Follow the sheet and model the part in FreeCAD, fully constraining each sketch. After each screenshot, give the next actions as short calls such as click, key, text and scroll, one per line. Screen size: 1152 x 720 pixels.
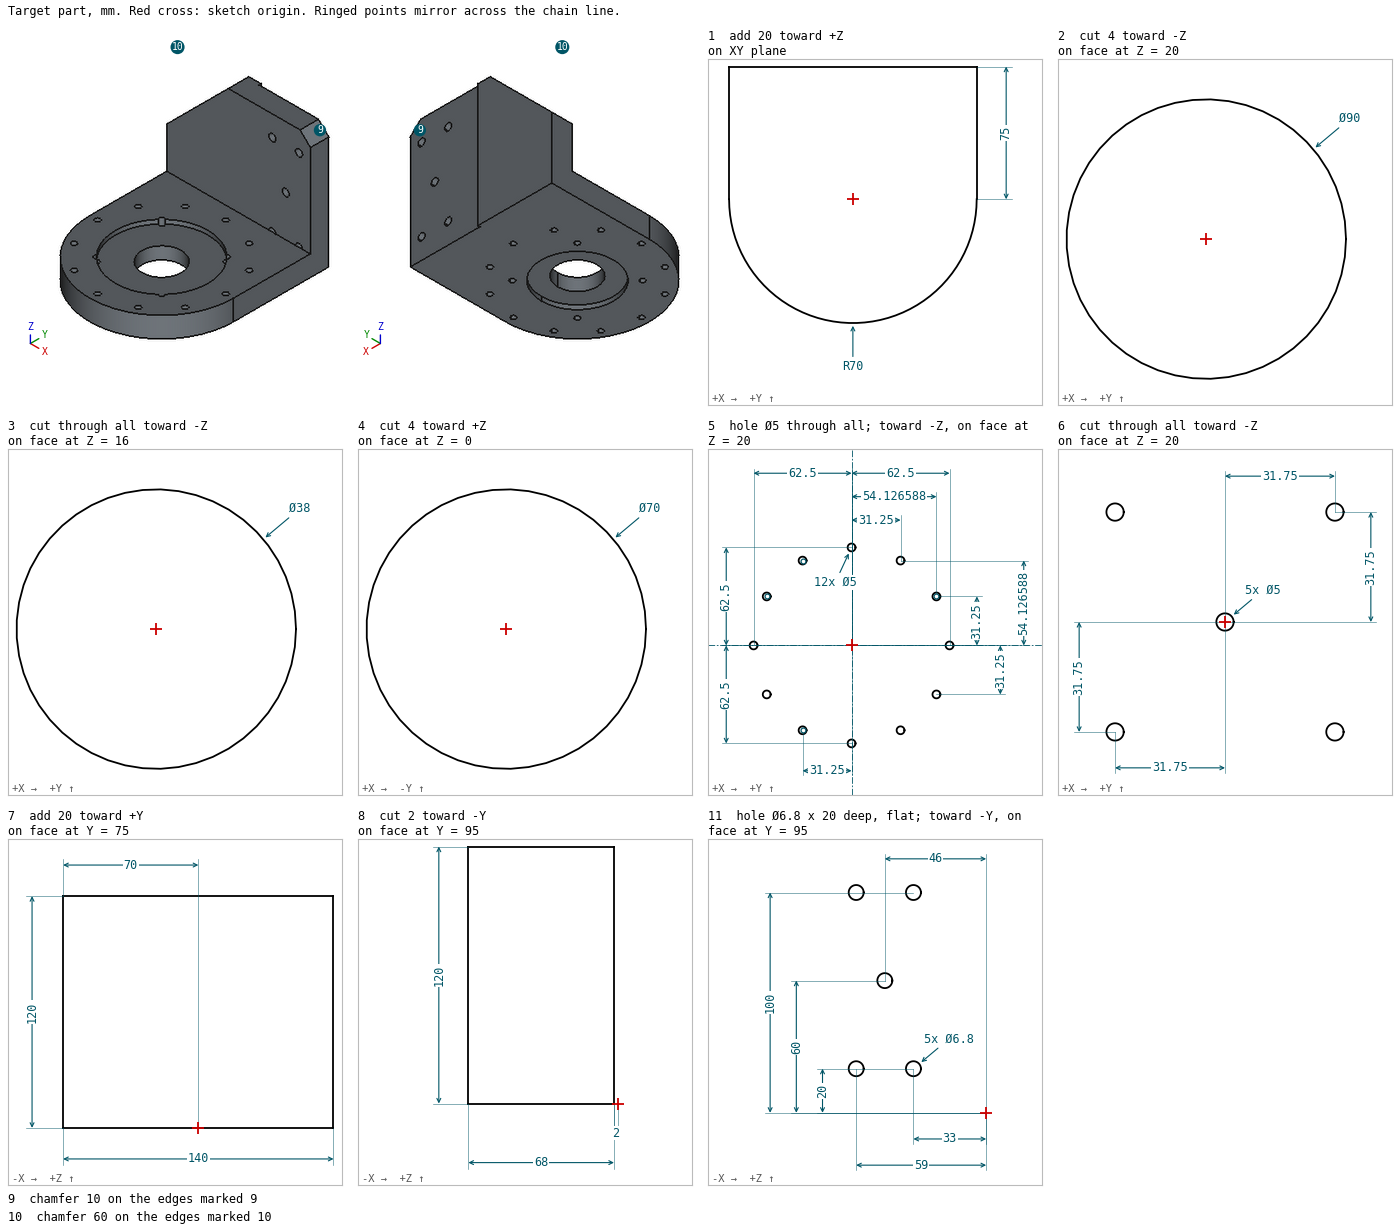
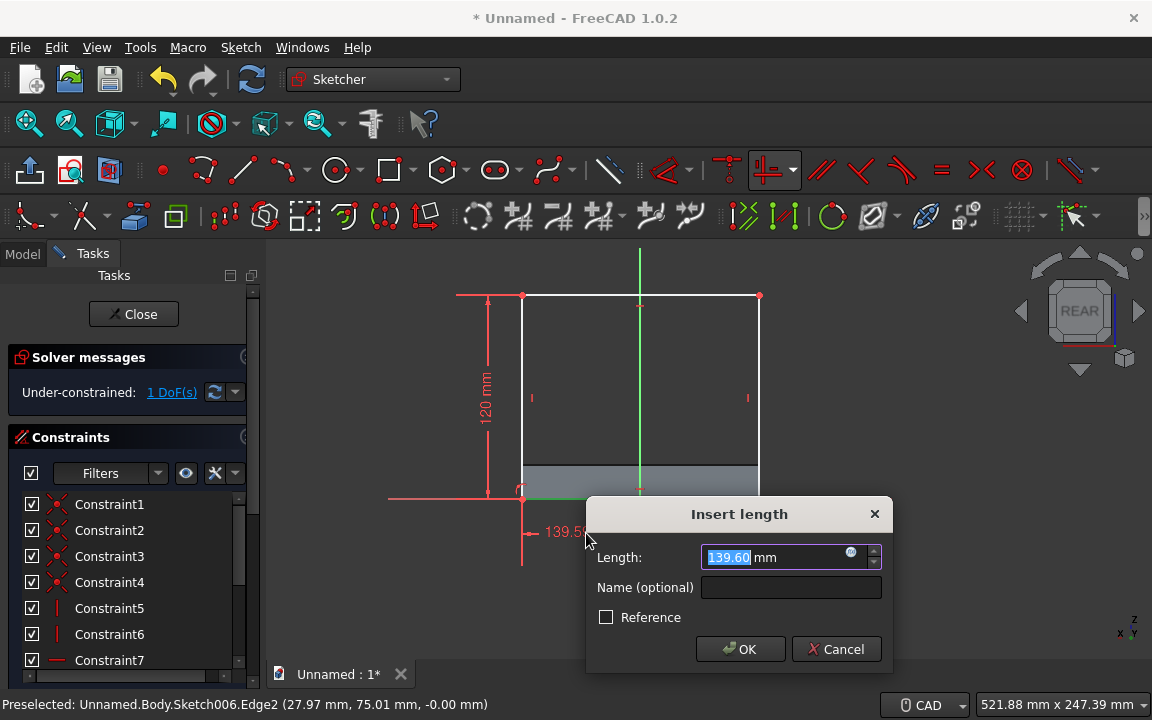
text(140)
key(Return)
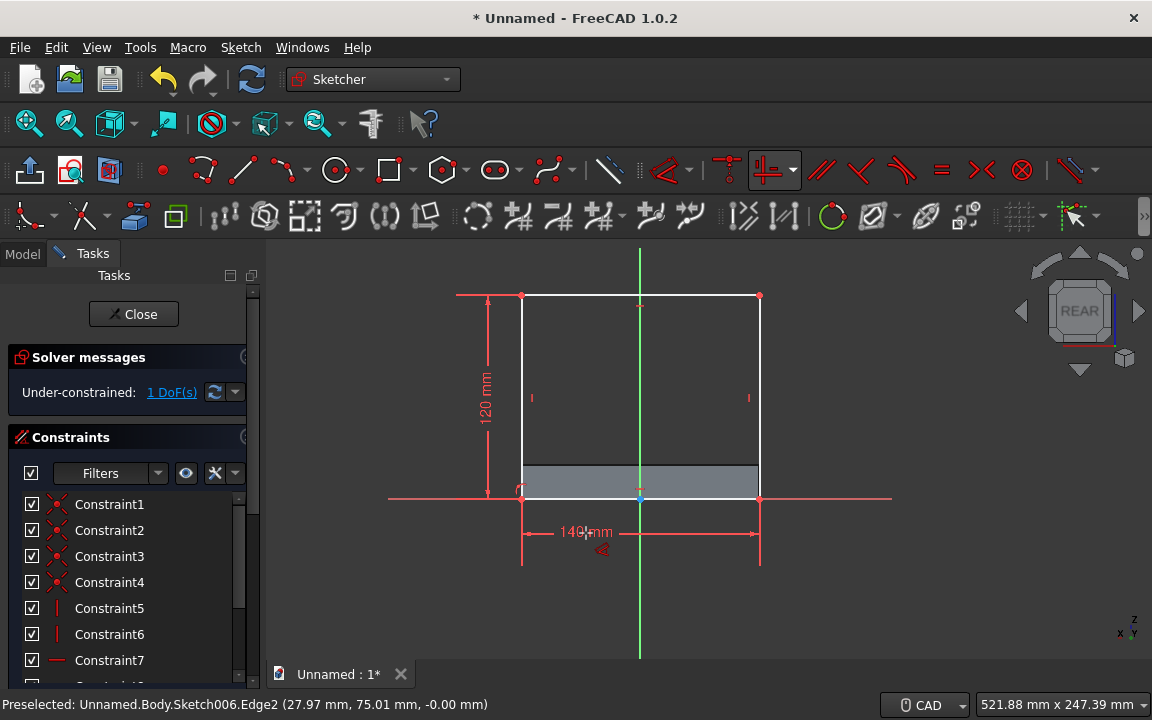
click(522, 295)
click(581, 557)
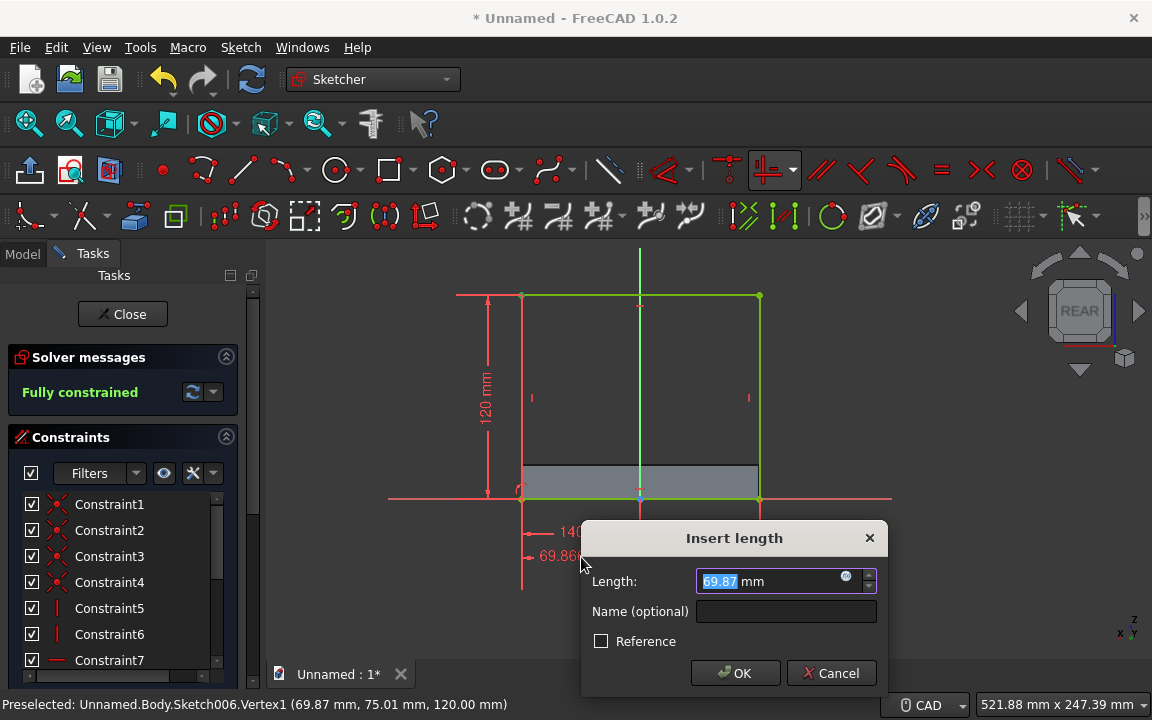
text(70)
key(Return)
key(Escape)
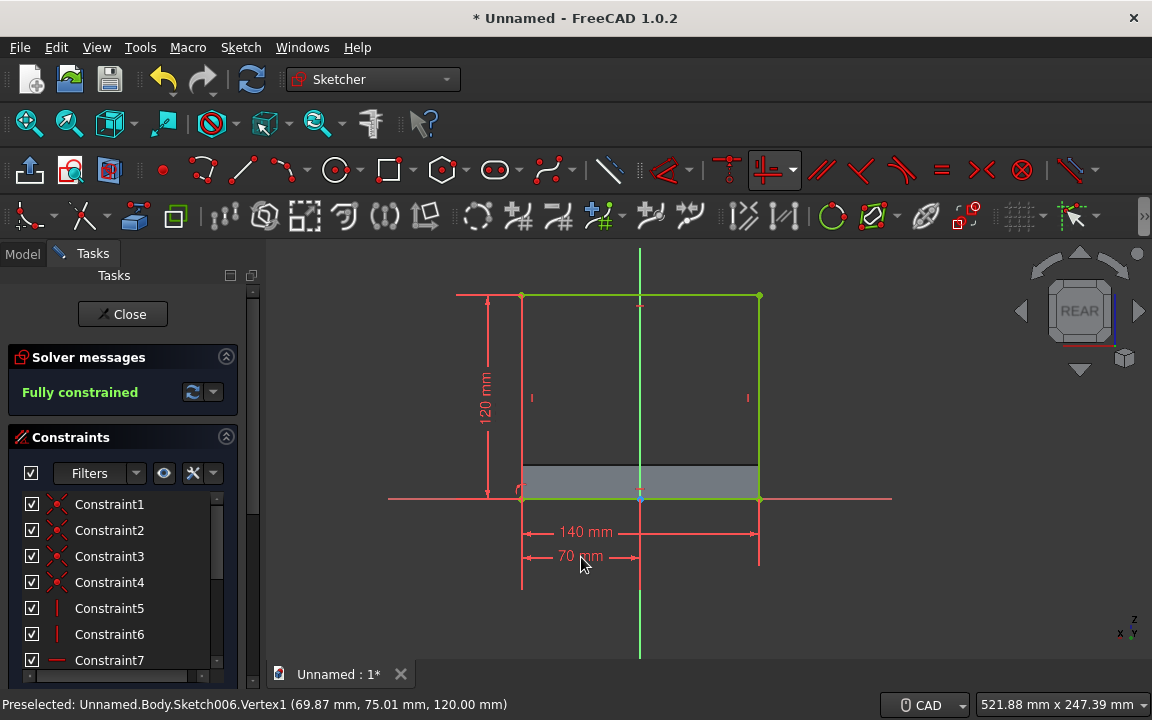
click(123, 314)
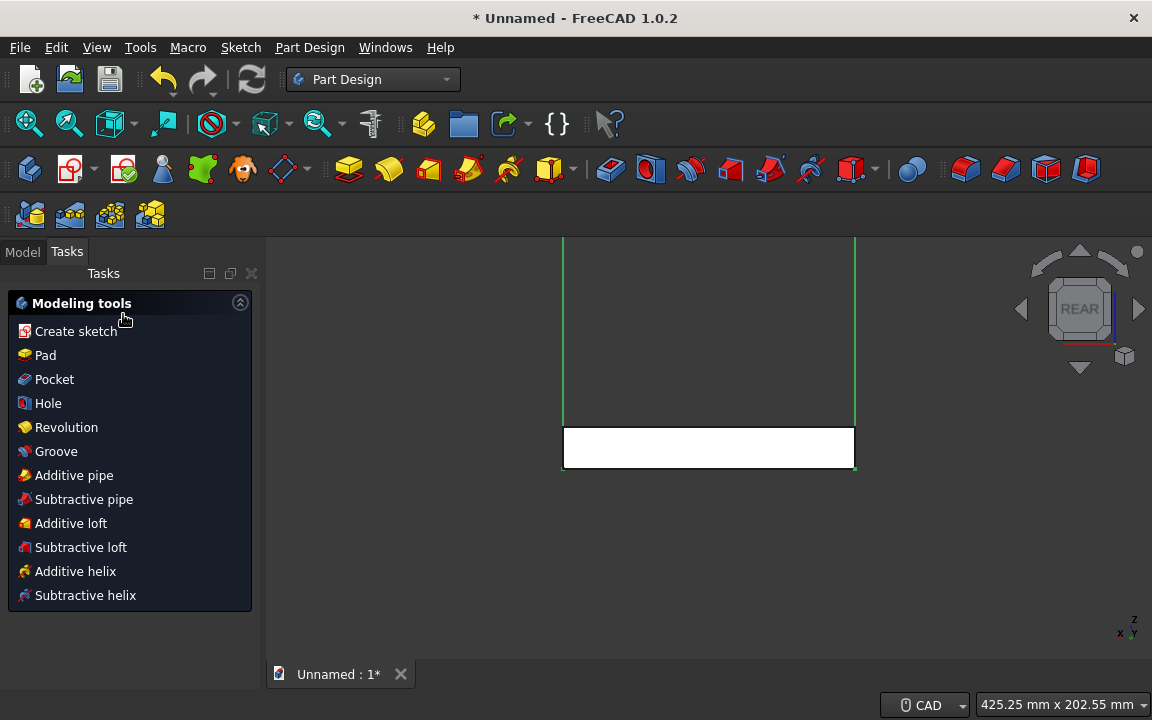
click(350, 170)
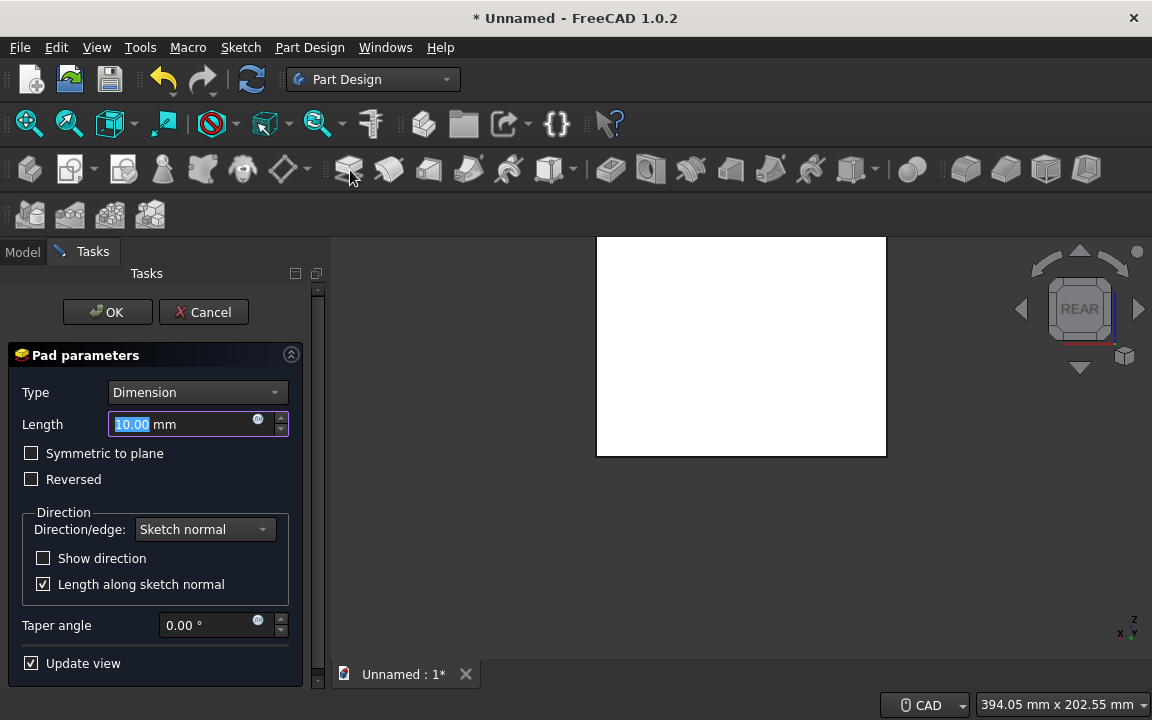
text(20)
key(Tab)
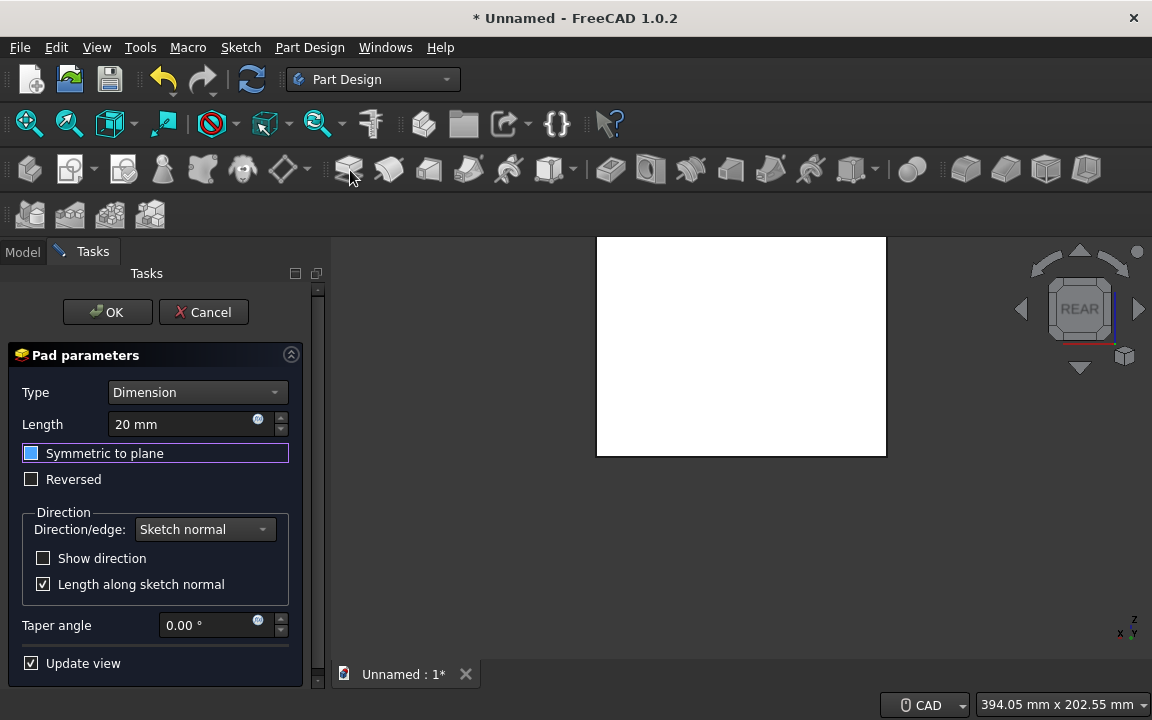
click(108, 312)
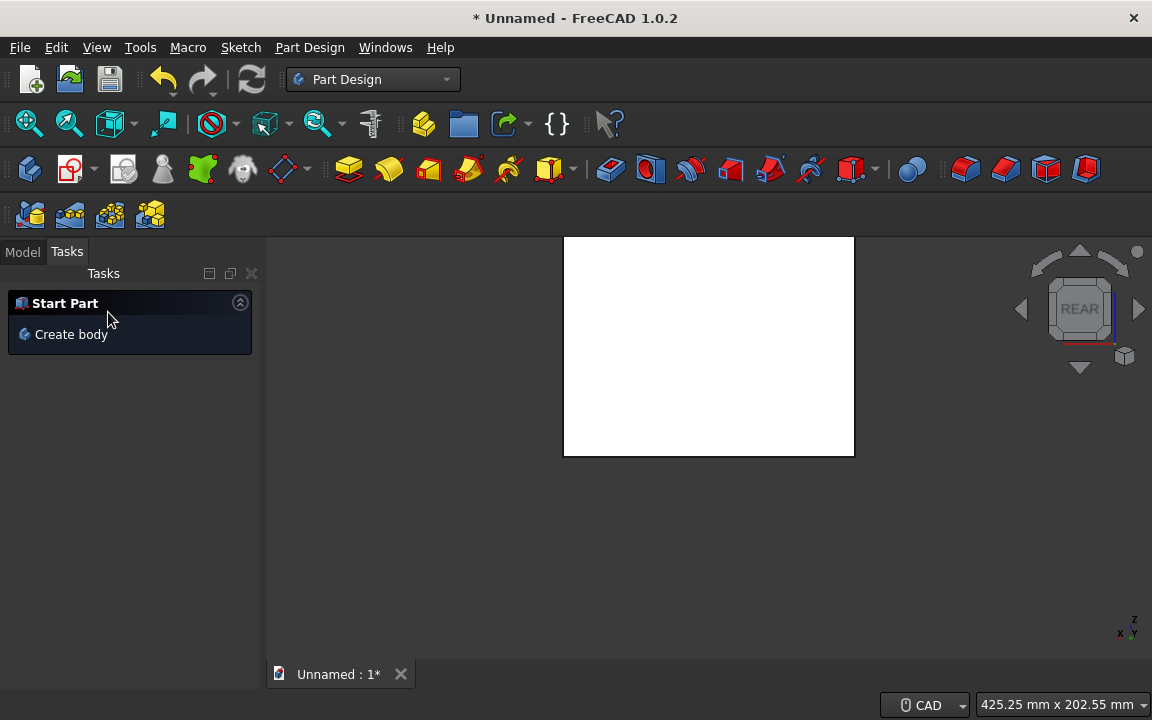
click(30, 124)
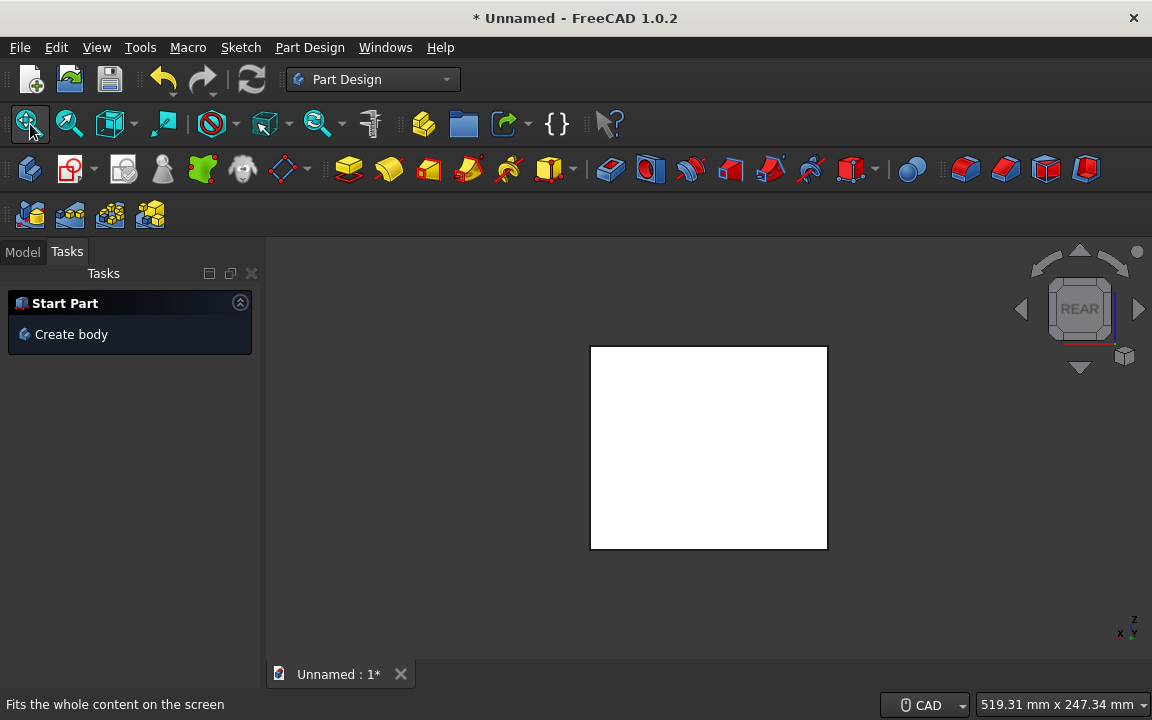
click(709, 447)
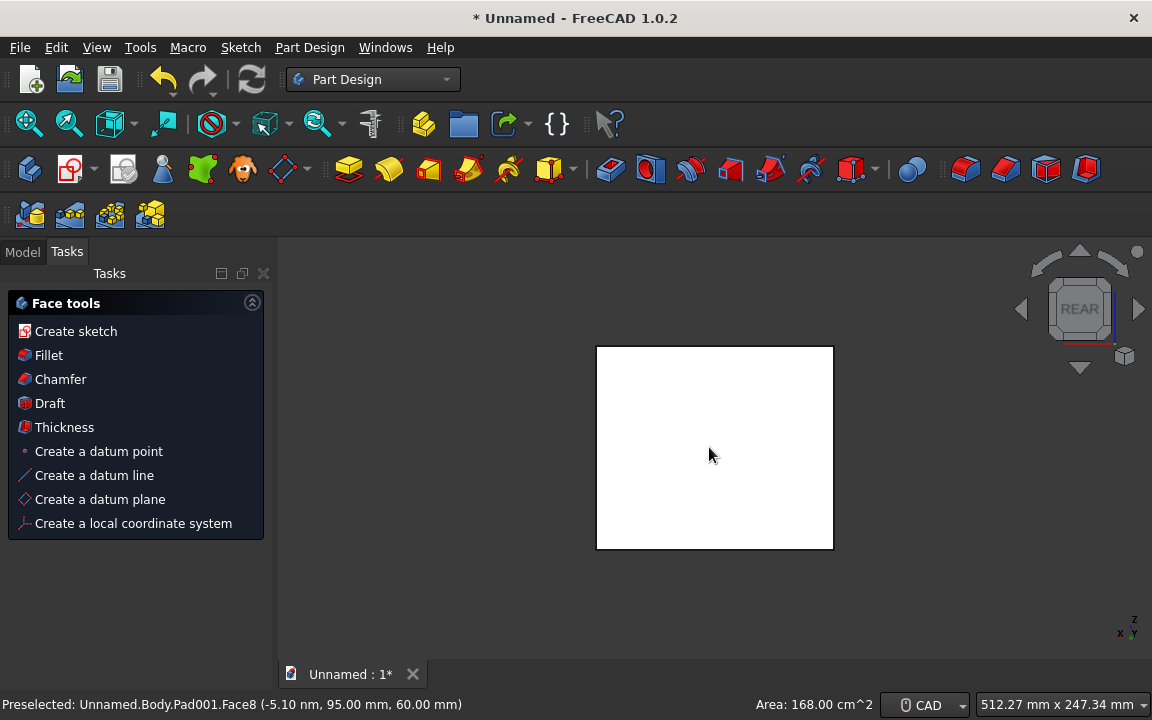
click(70, 170)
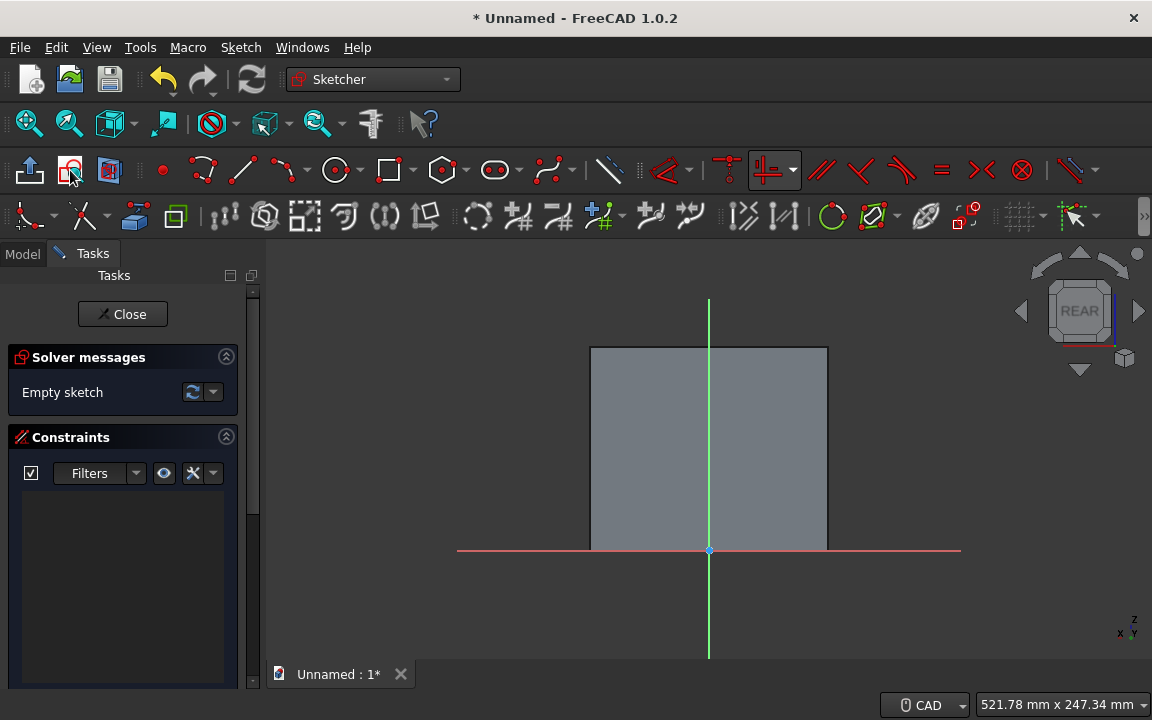
key(g)
key(r)